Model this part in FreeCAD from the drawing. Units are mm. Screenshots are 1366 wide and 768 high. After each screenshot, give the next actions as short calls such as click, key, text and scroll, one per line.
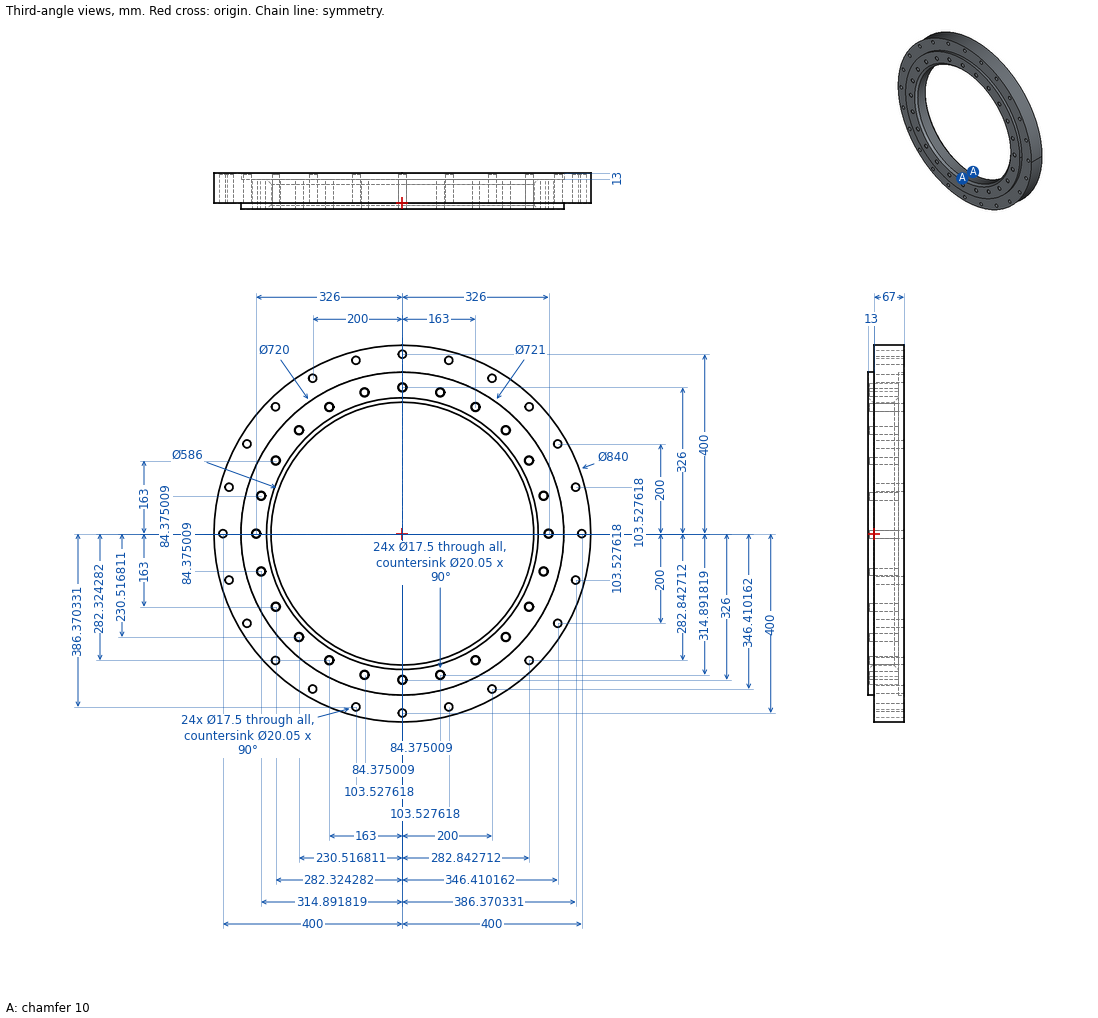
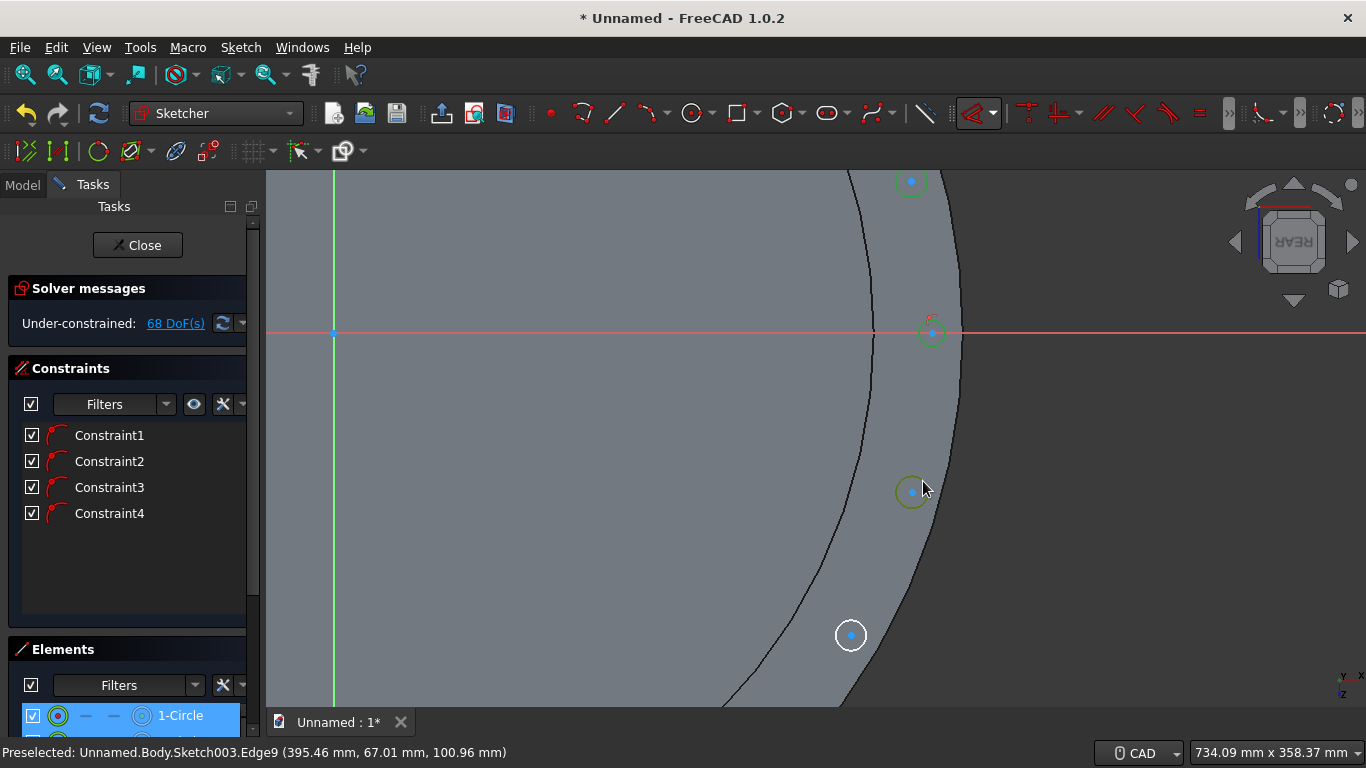
click(862, 625)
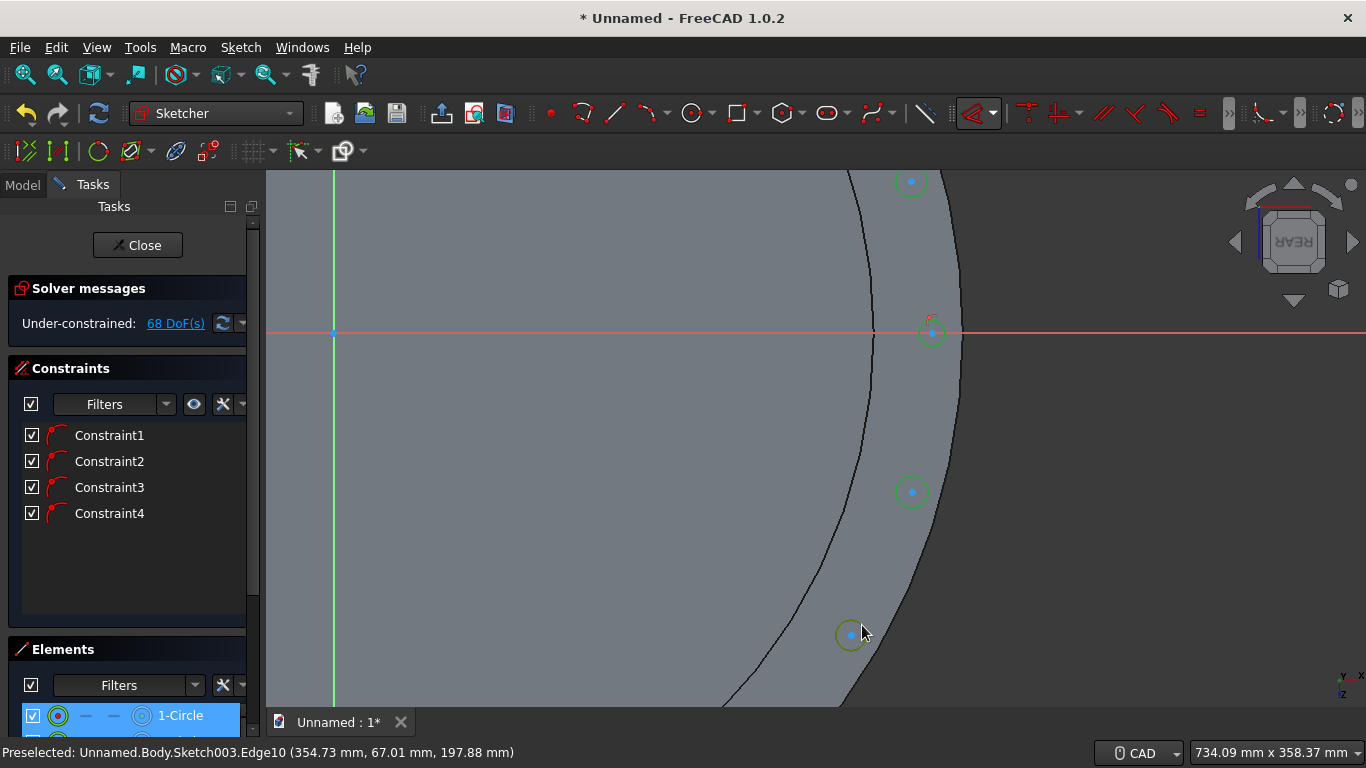
scroll(926, 484, down, 6)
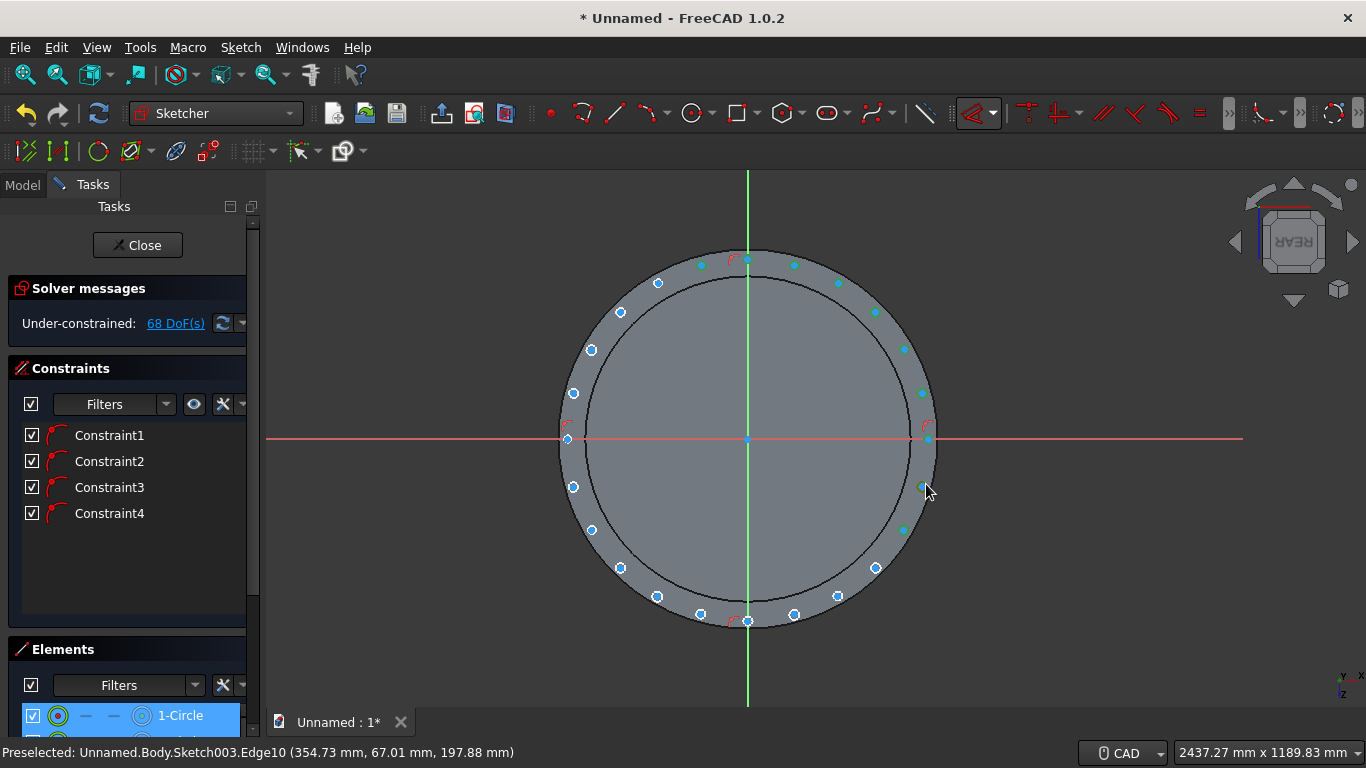
scroll(879, 565, up, 6)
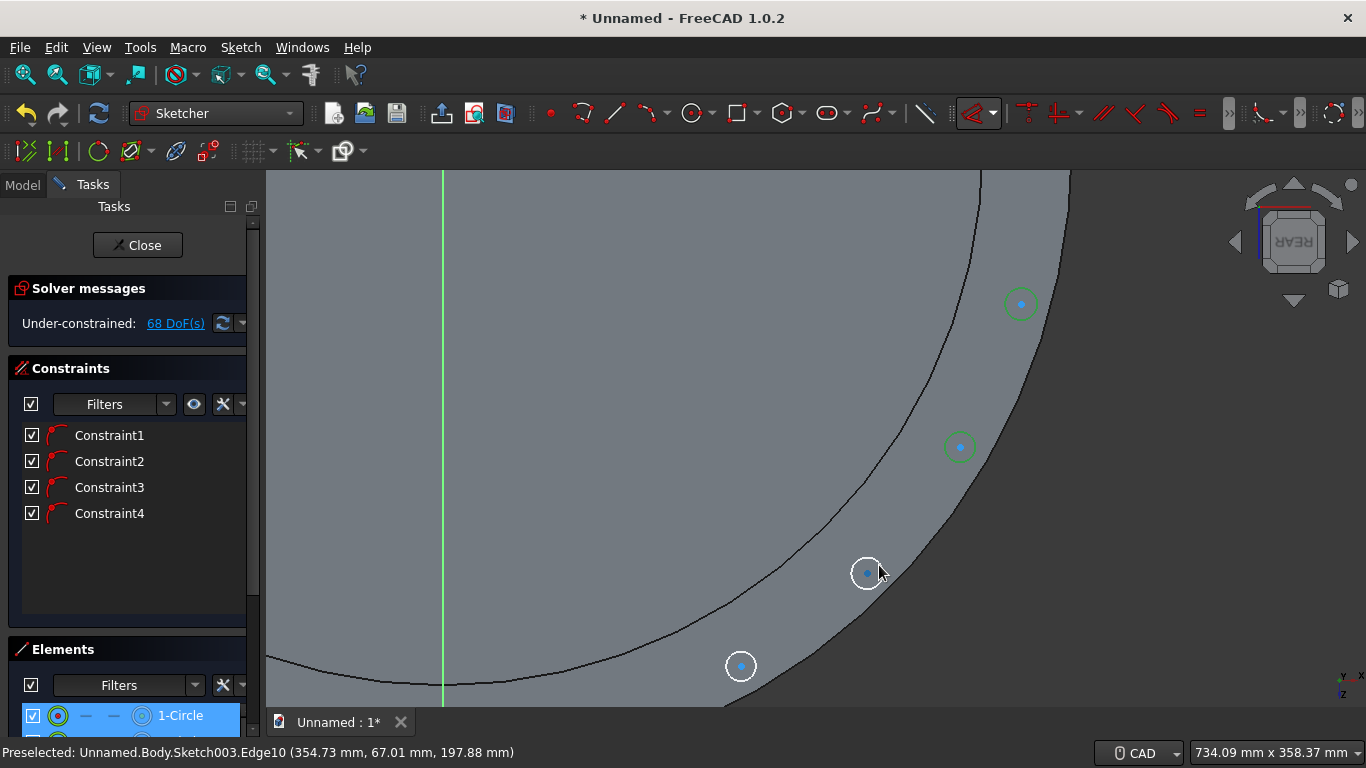
click(878, 562)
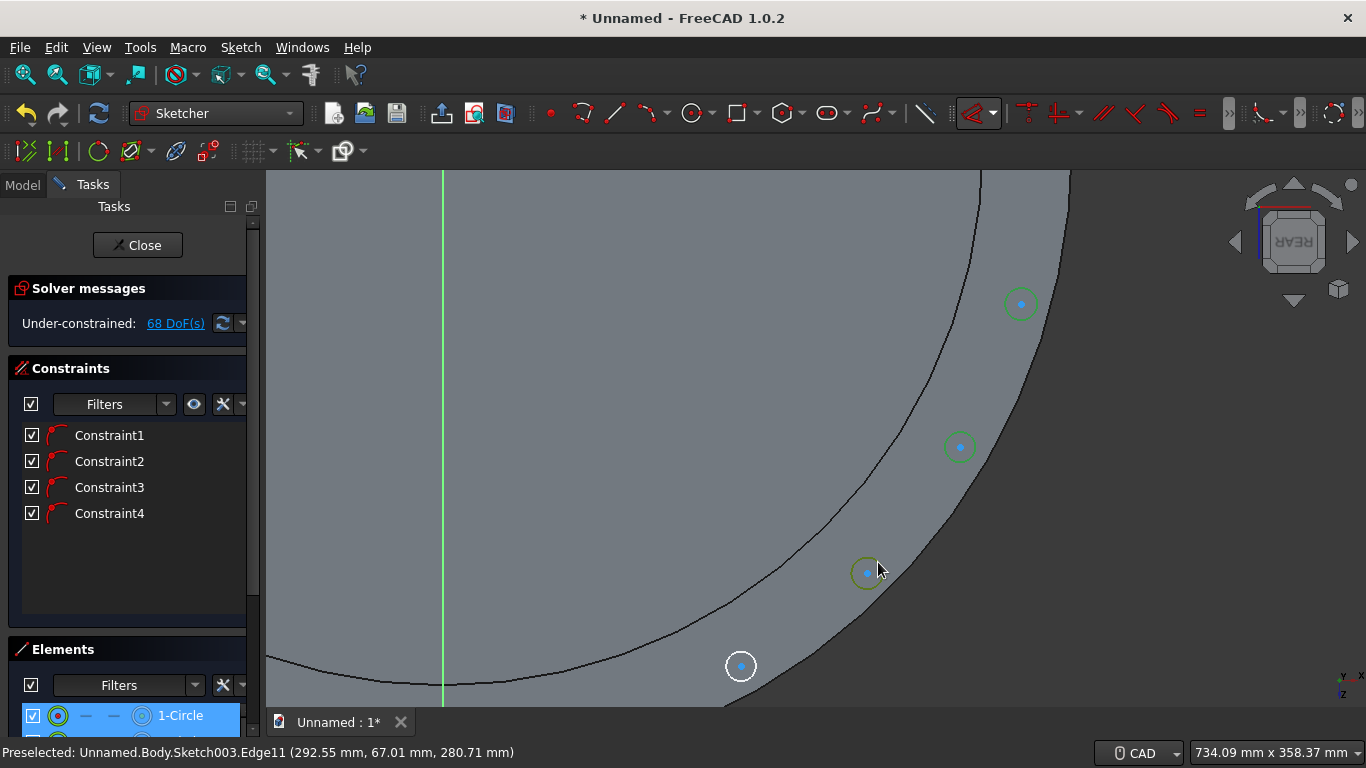
click(751, 656)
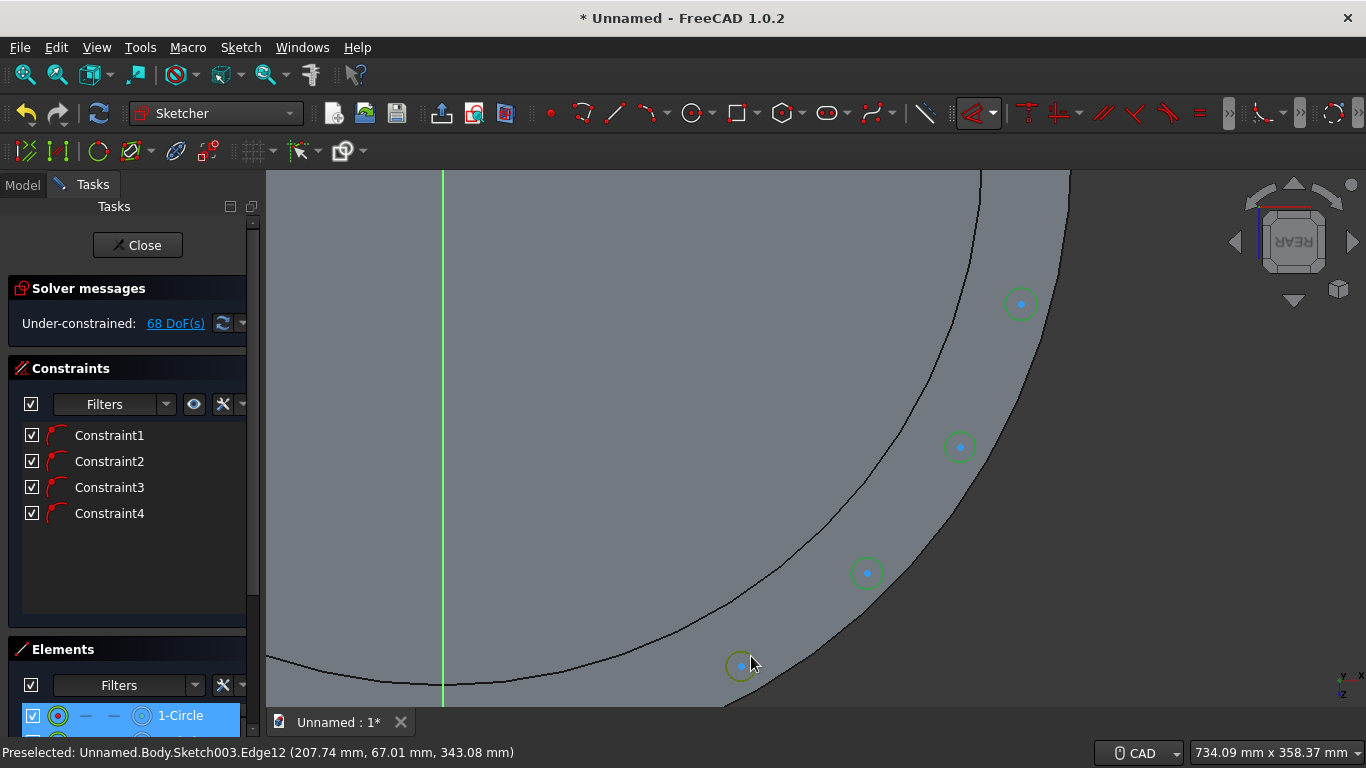
scroll(879, 565, down, 6)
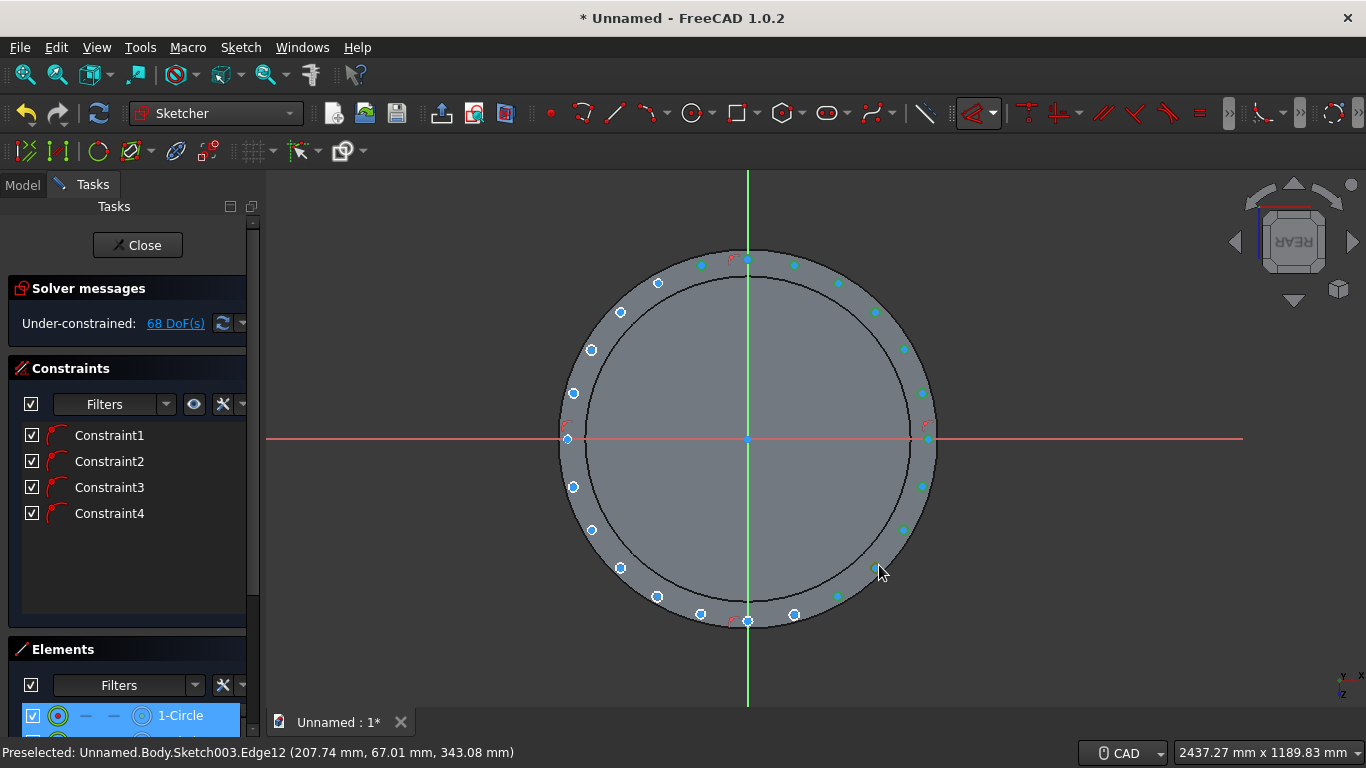
scroll(798, 611, up, 6)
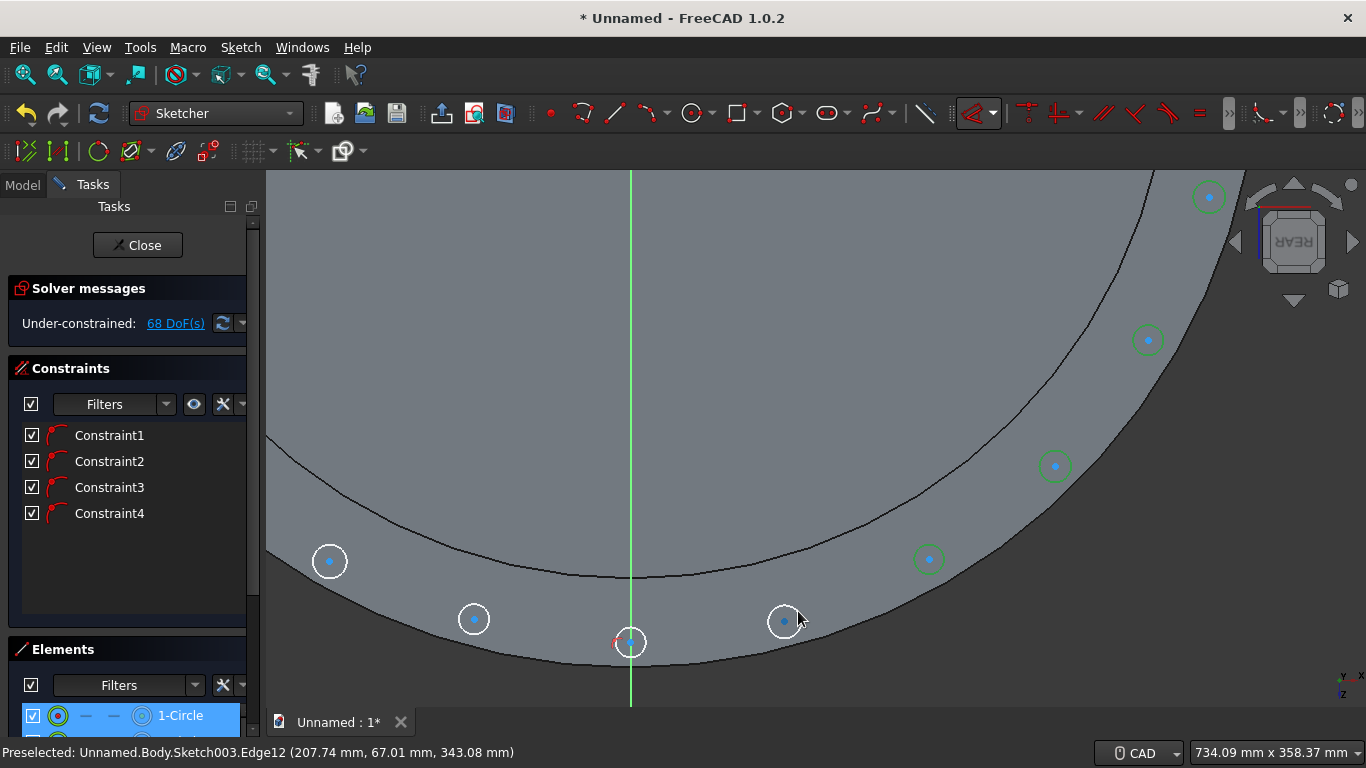
click(796, 610)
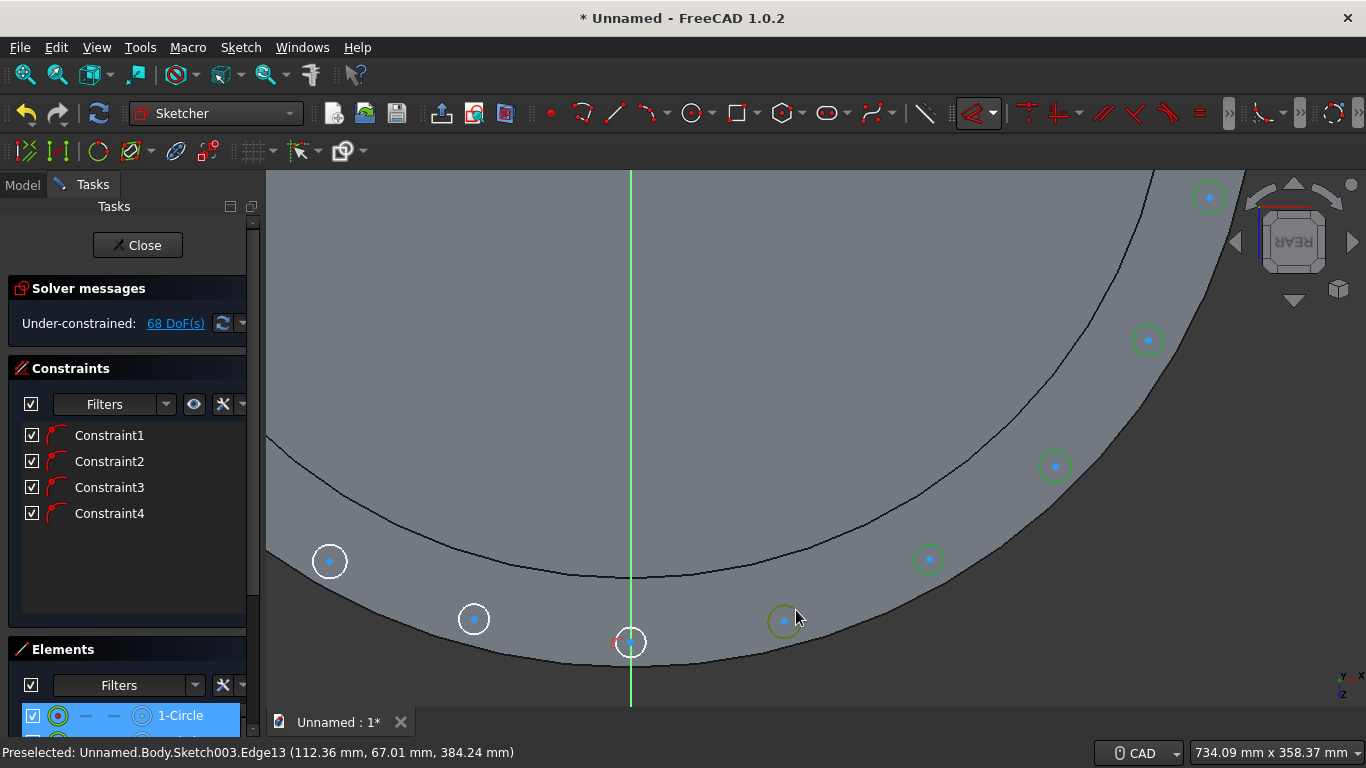
scroll(641, 632, up, 2)